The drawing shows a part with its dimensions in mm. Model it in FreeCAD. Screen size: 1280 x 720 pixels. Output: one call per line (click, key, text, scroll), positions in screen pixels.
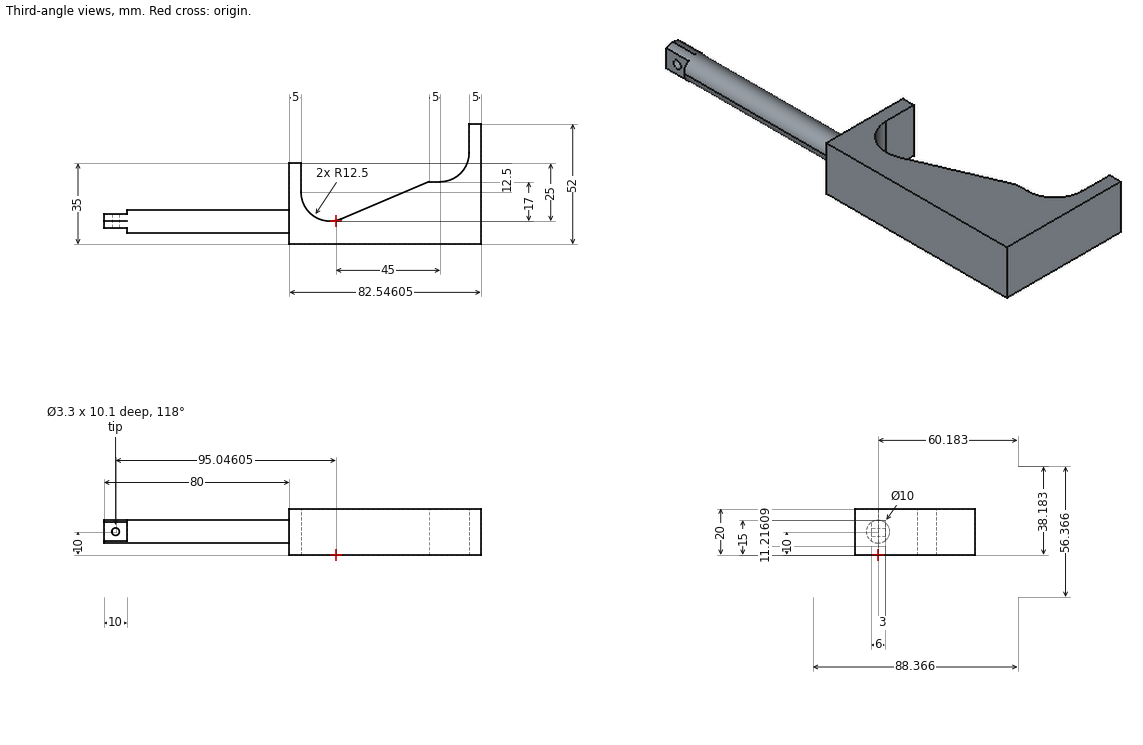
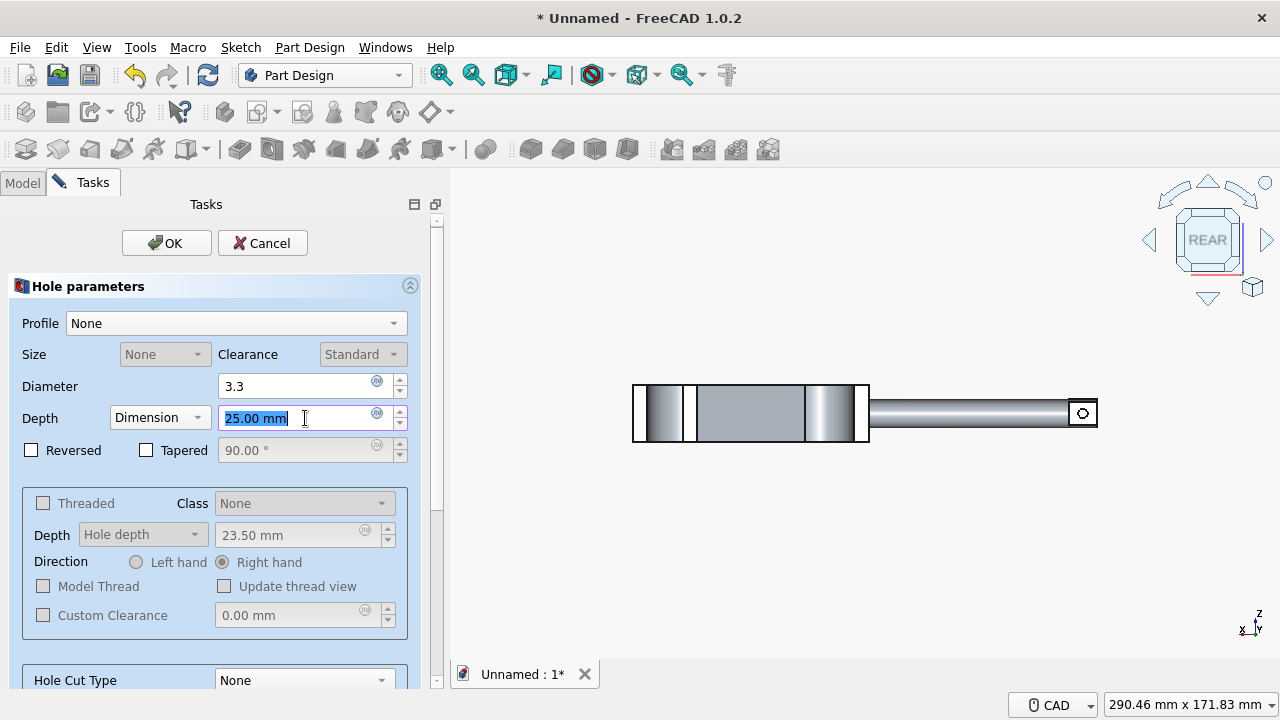
text(10.1)
key(Tab)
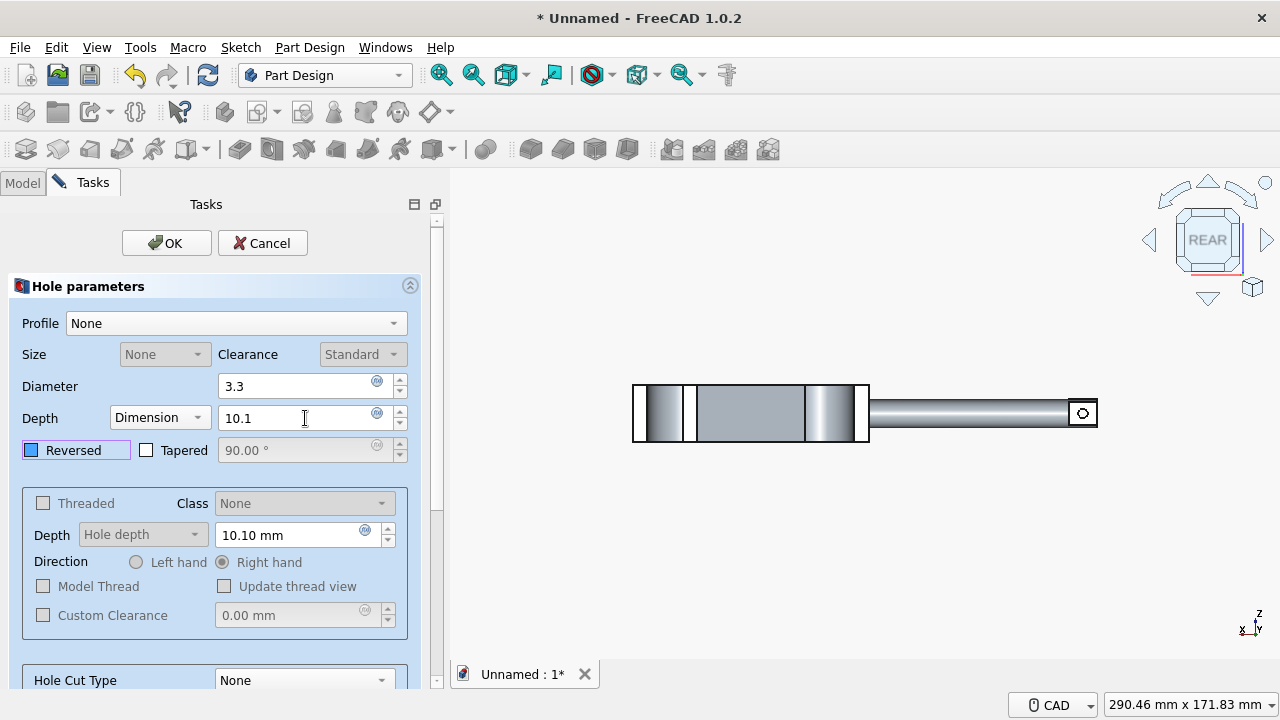
click(167, 243)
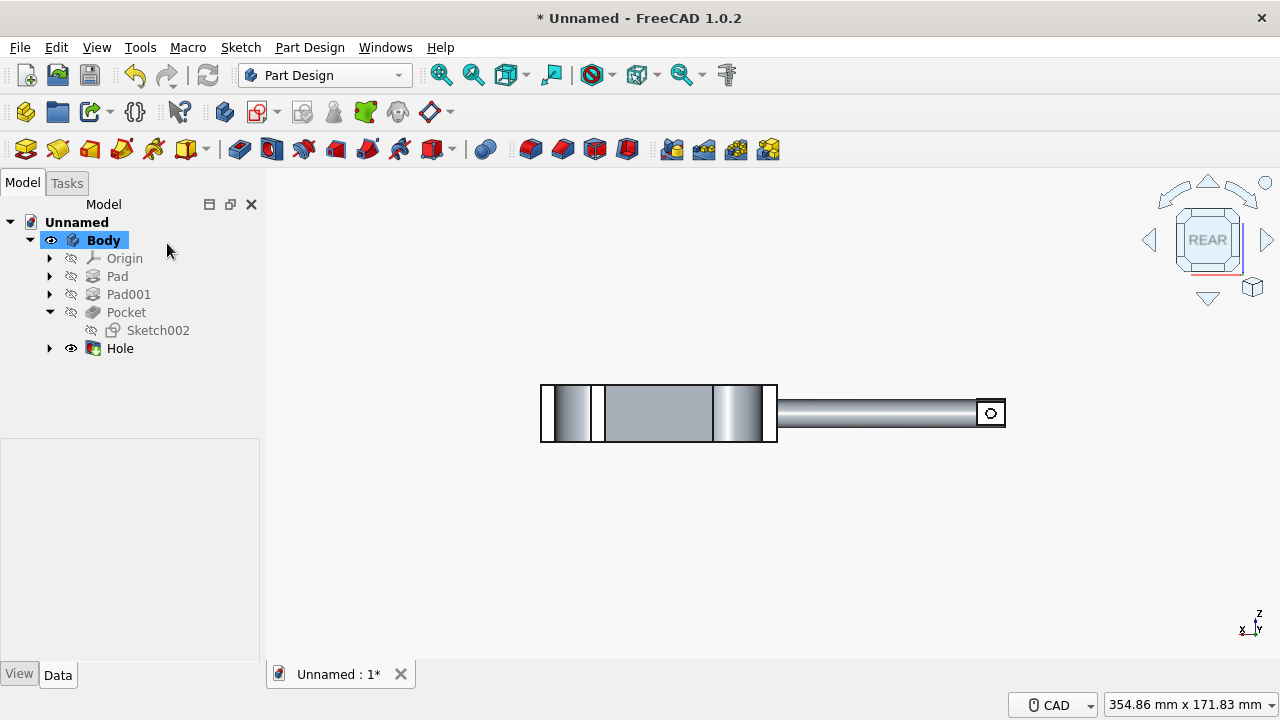
key(0)